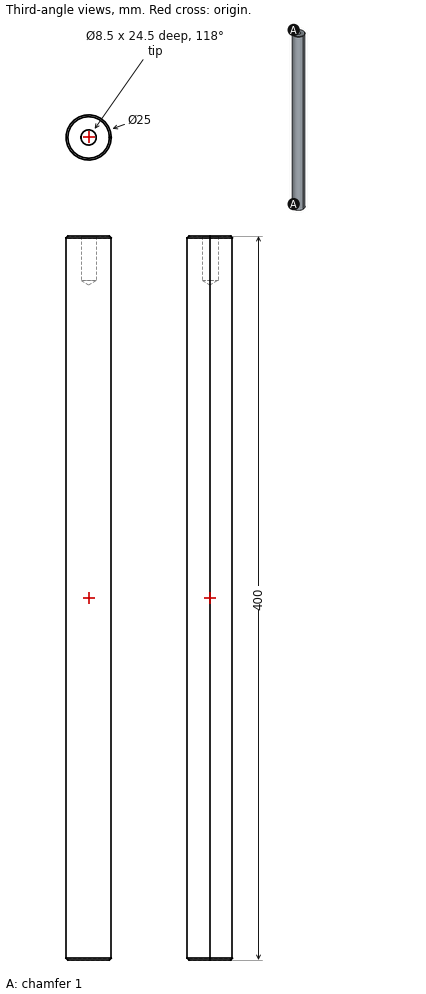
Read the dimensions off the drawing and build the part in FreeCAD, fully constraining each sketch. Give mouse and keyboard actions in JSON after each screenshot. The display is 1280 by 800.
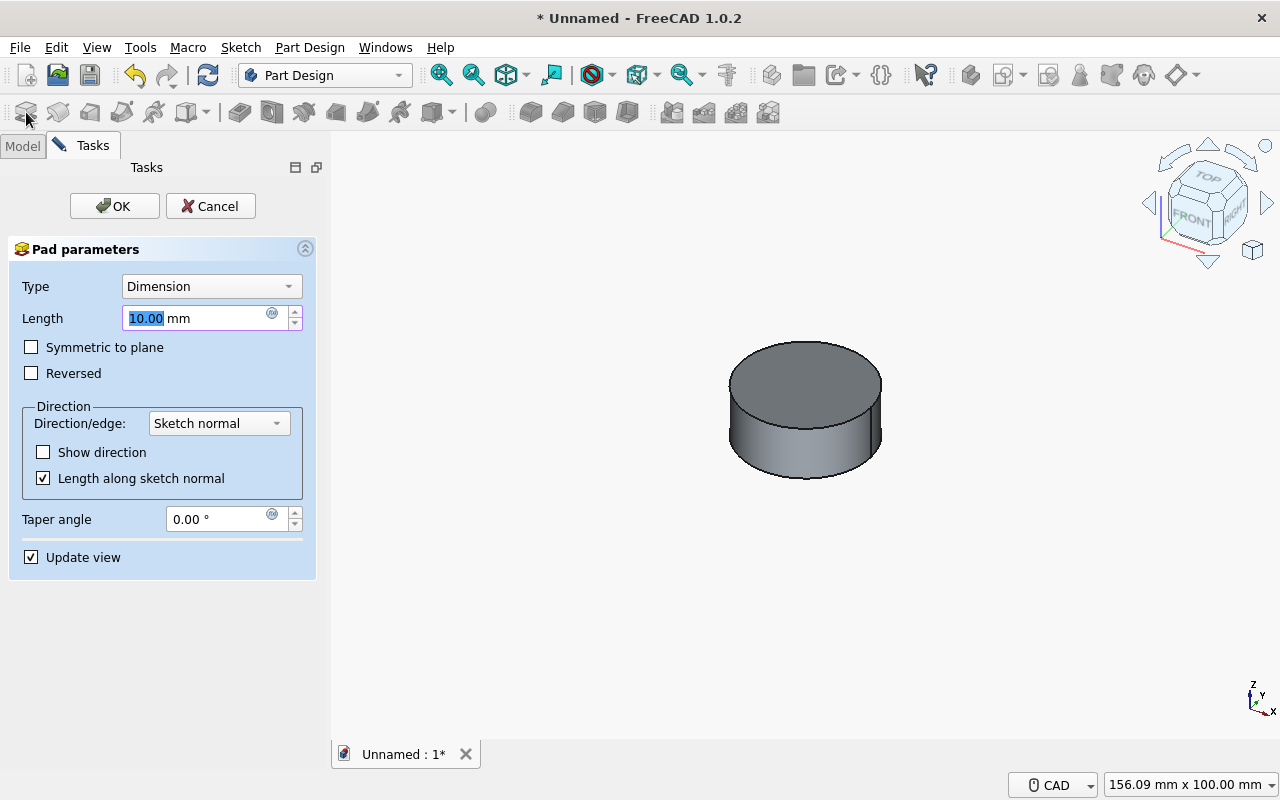
{"action": "type", "text": "400"}
{"action": "key", "text": "Tab"}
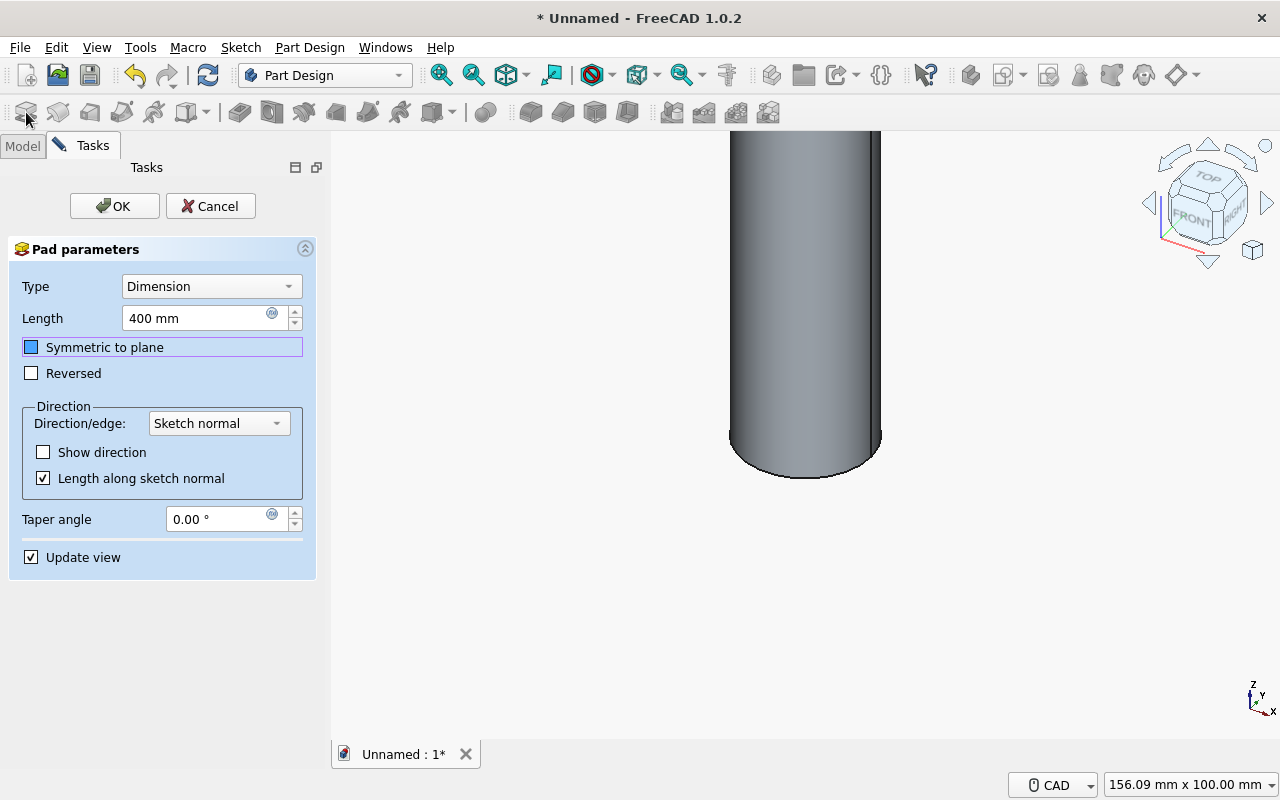
{"action": "left_click", "coordinate": [30, 347]}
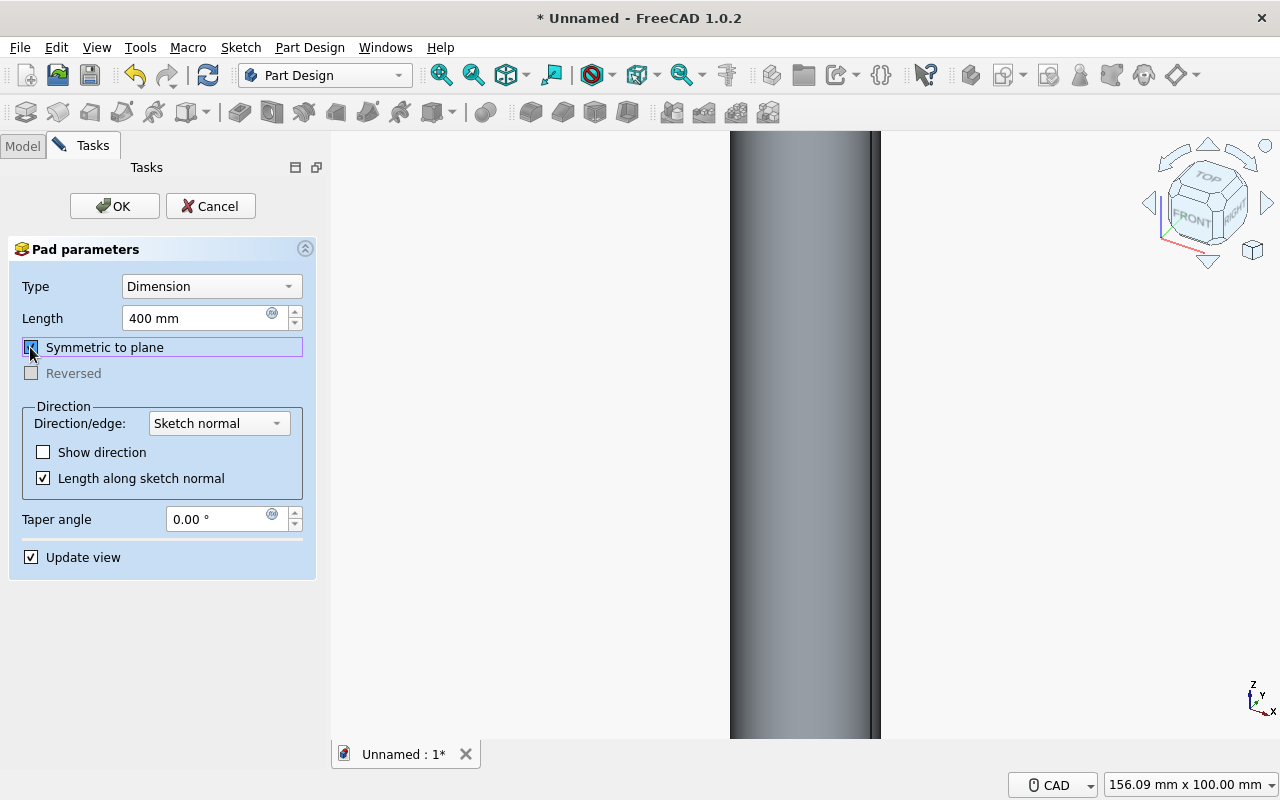
{"action": "left_click", "coordinate": [115, 206]}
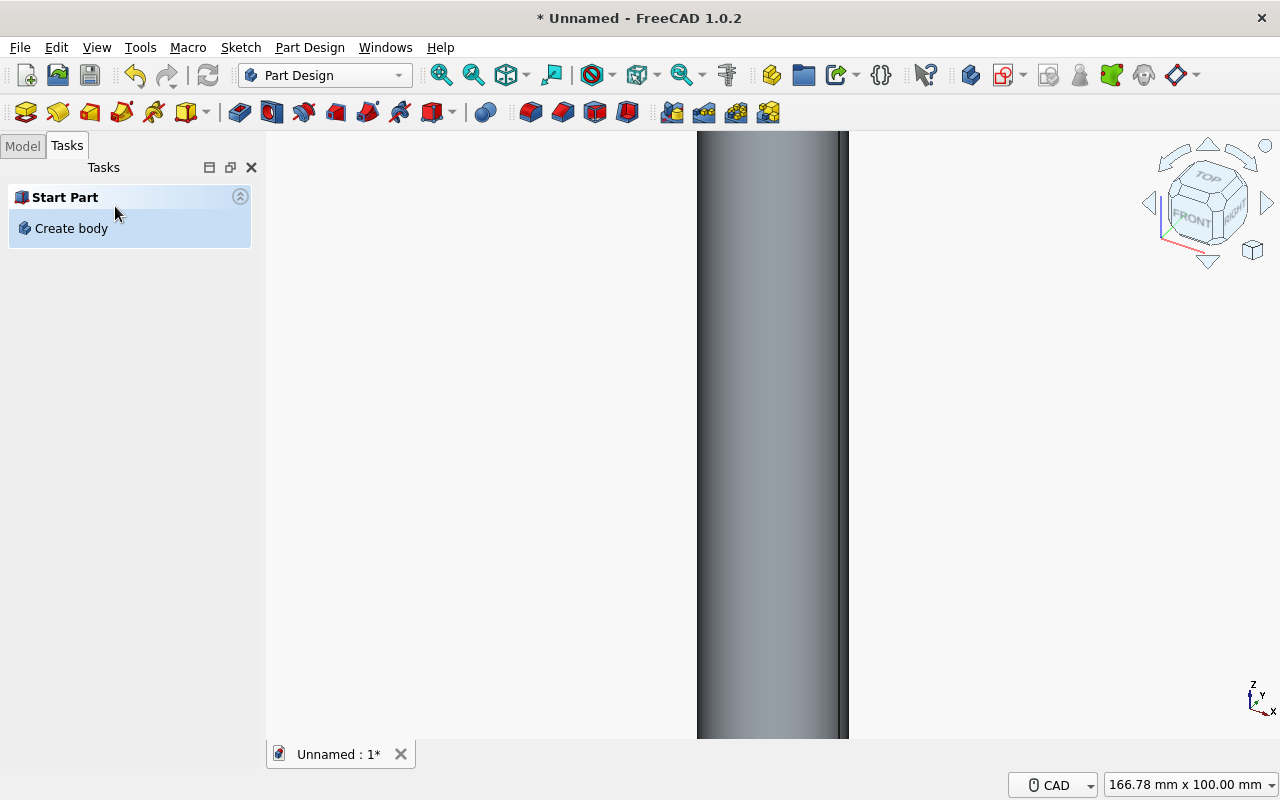
{"action": "left_click", "coordinate": [442, 76]}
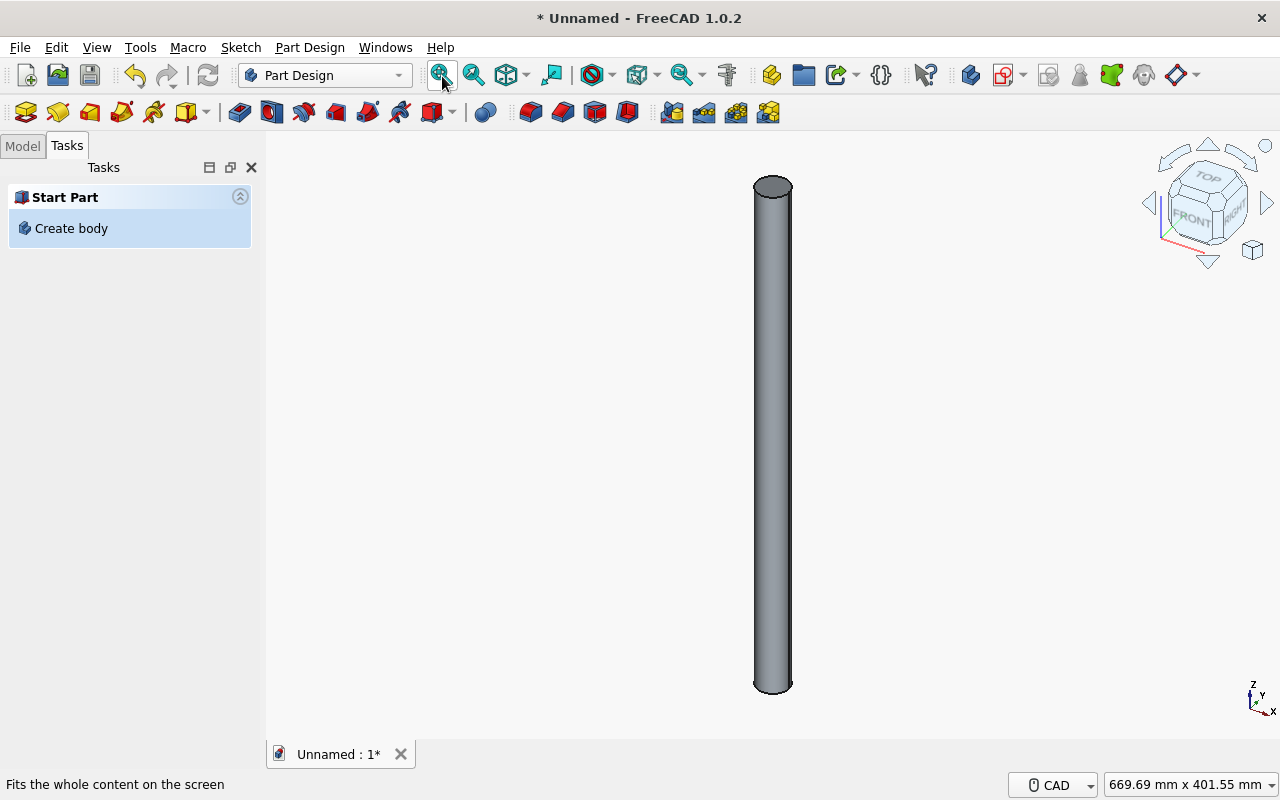
{"action": "left_click", "coordinate": [757, 181]}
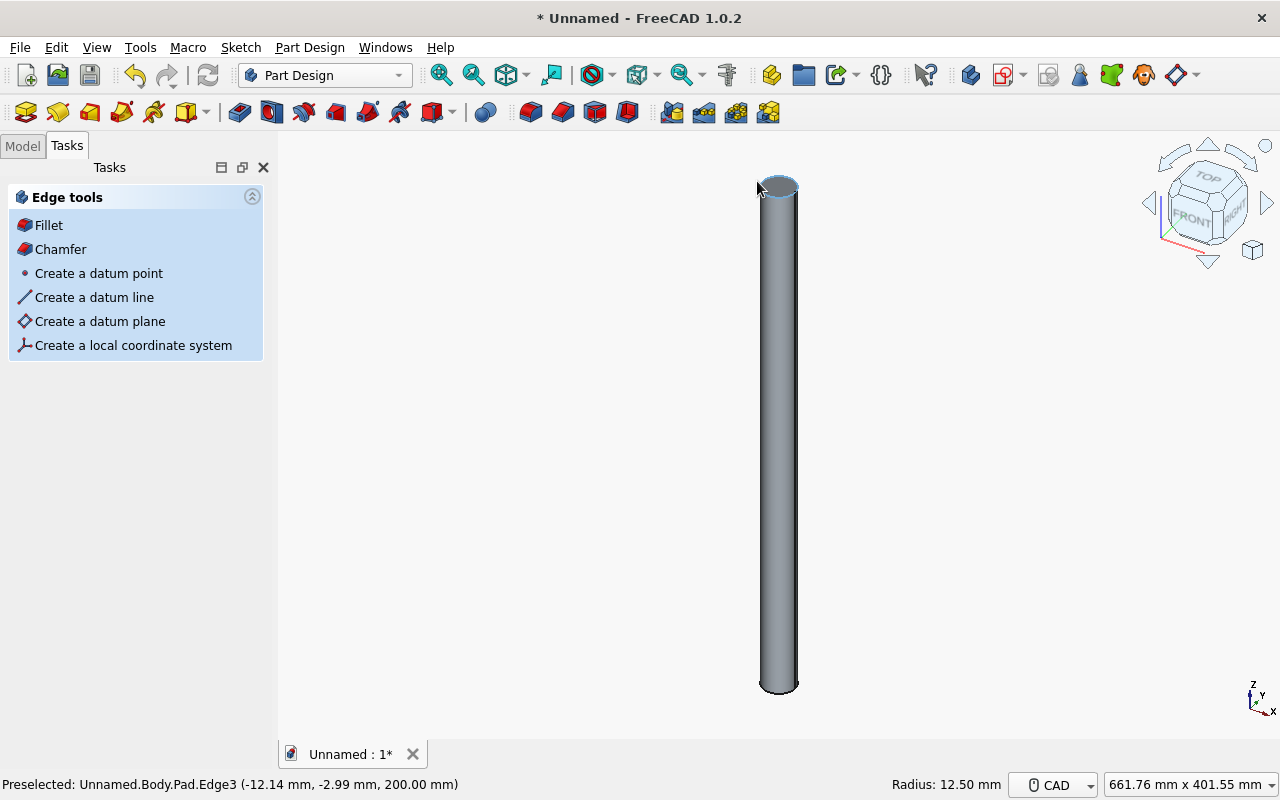
{"action": "key", "text": "0"}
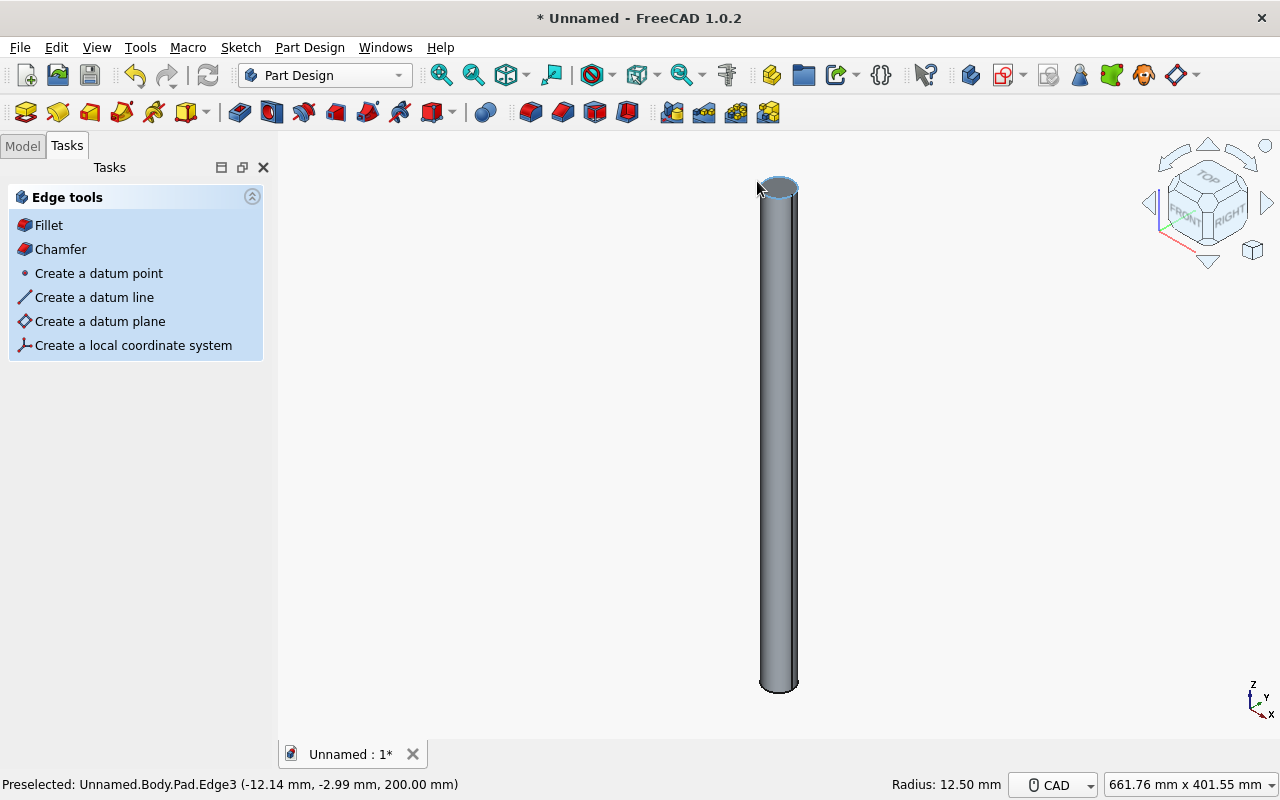
{"action": "left_click", "coordinate": [762, 686], "text": "ctrl"}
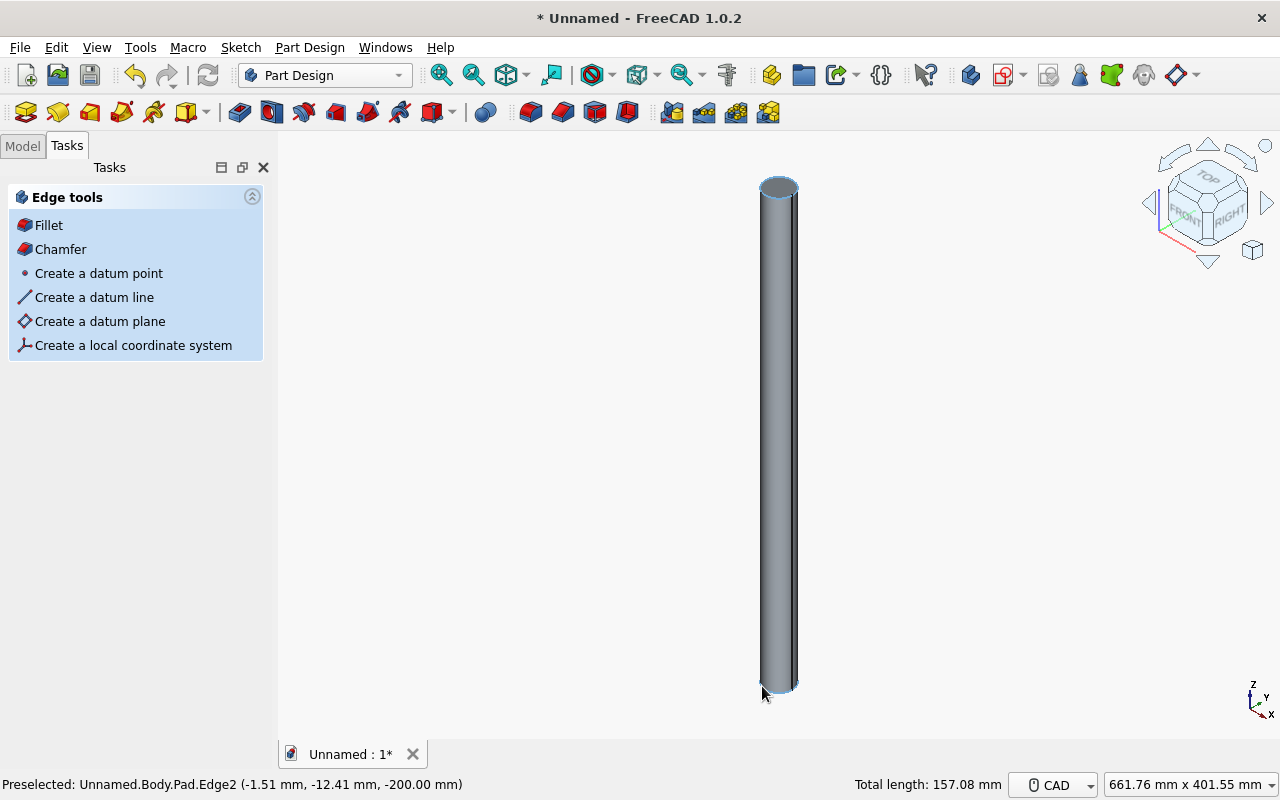
{"action": "left_click", "coordinate": [564, 112]}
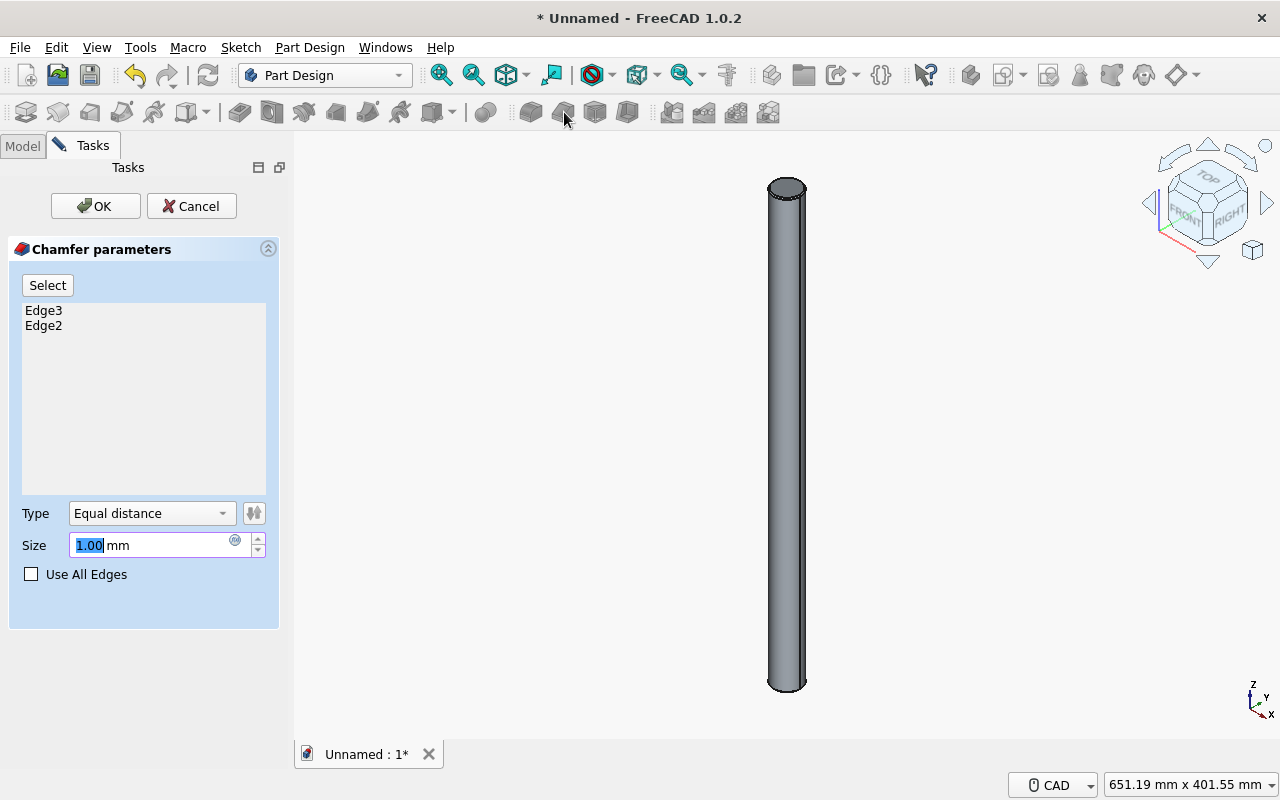
{"action": "type", "text": "1"}
{"action": "key", "text": "Tab"}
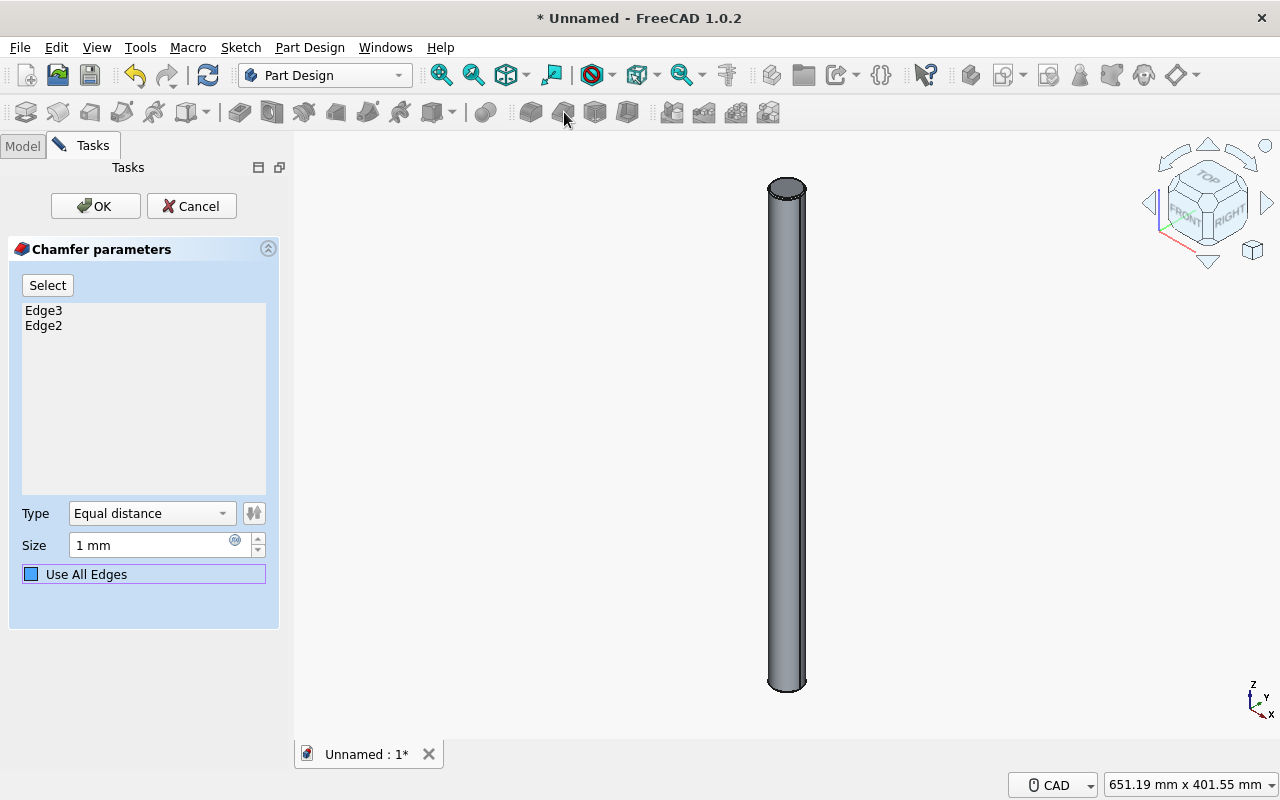
{"action": "left_click", "coordinate": [96, 206]}